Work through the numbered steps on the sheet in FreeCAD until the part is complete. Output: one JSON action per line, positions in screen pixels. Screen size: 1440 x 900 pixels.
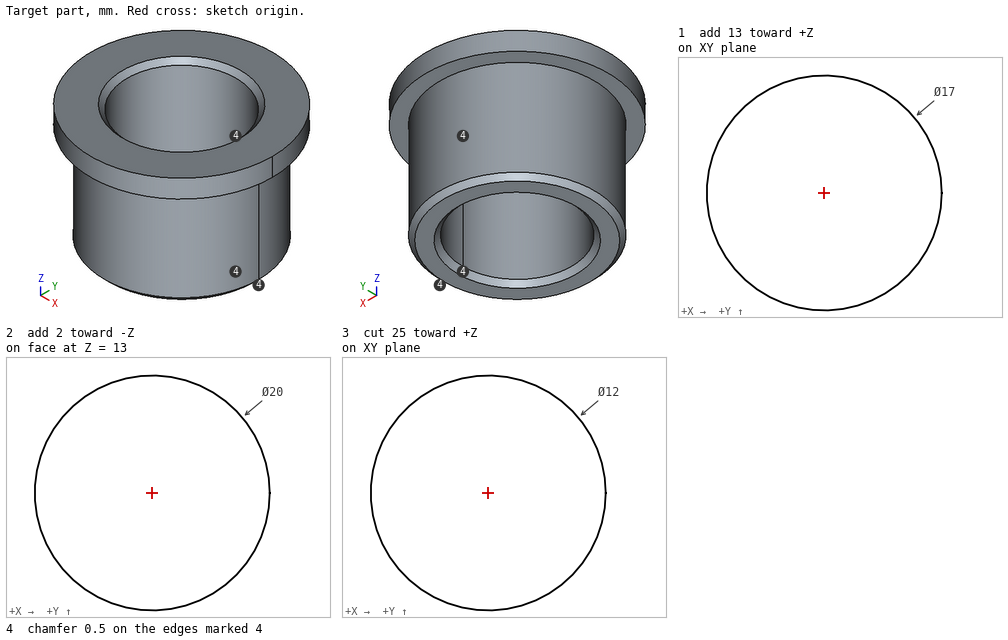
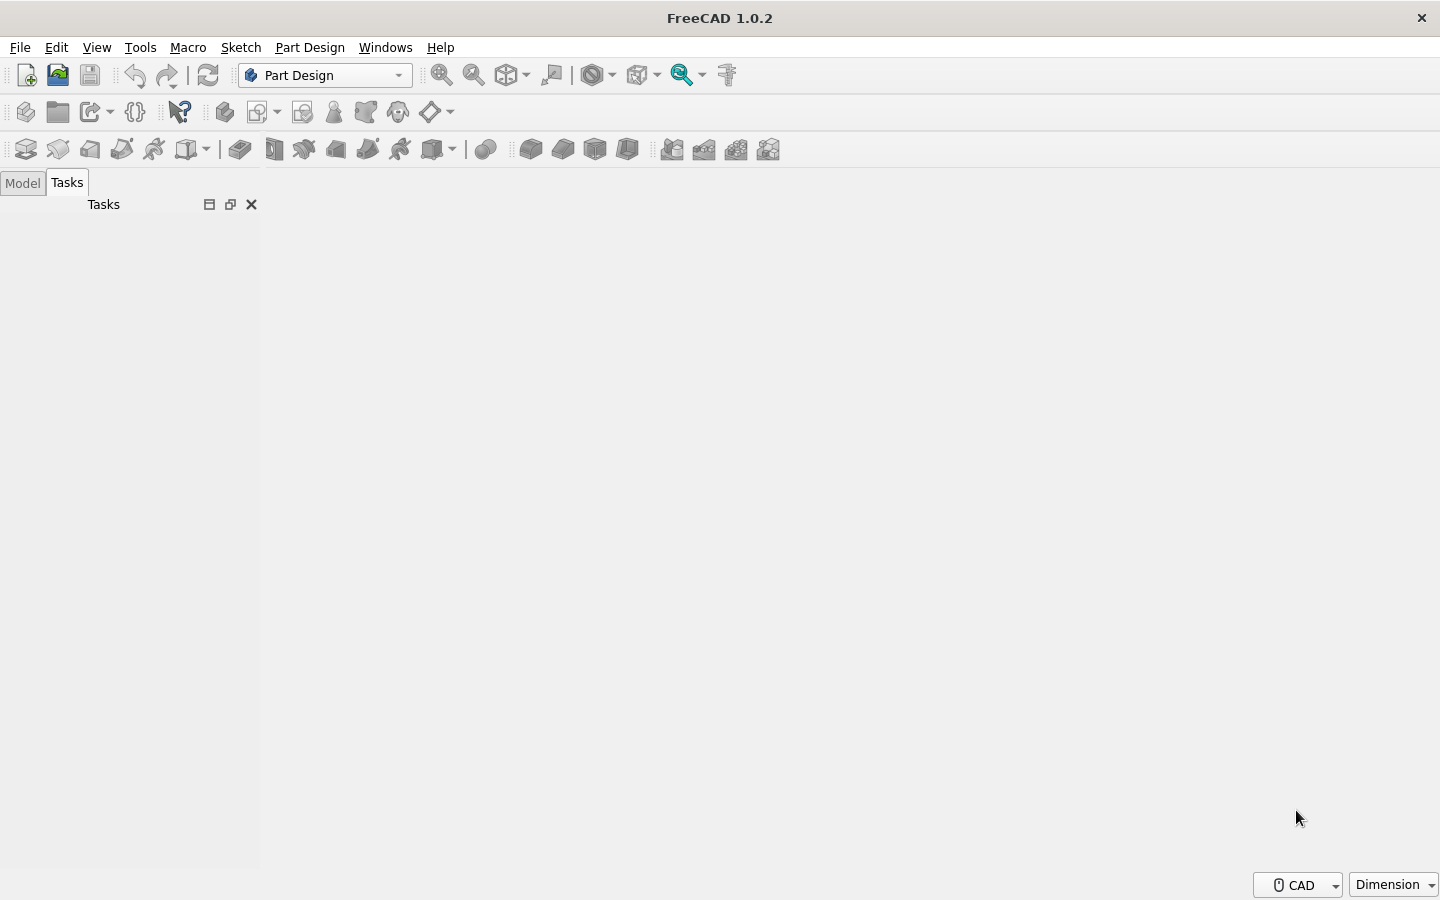
{"action": "left_click", "coordinate": [950, 76]}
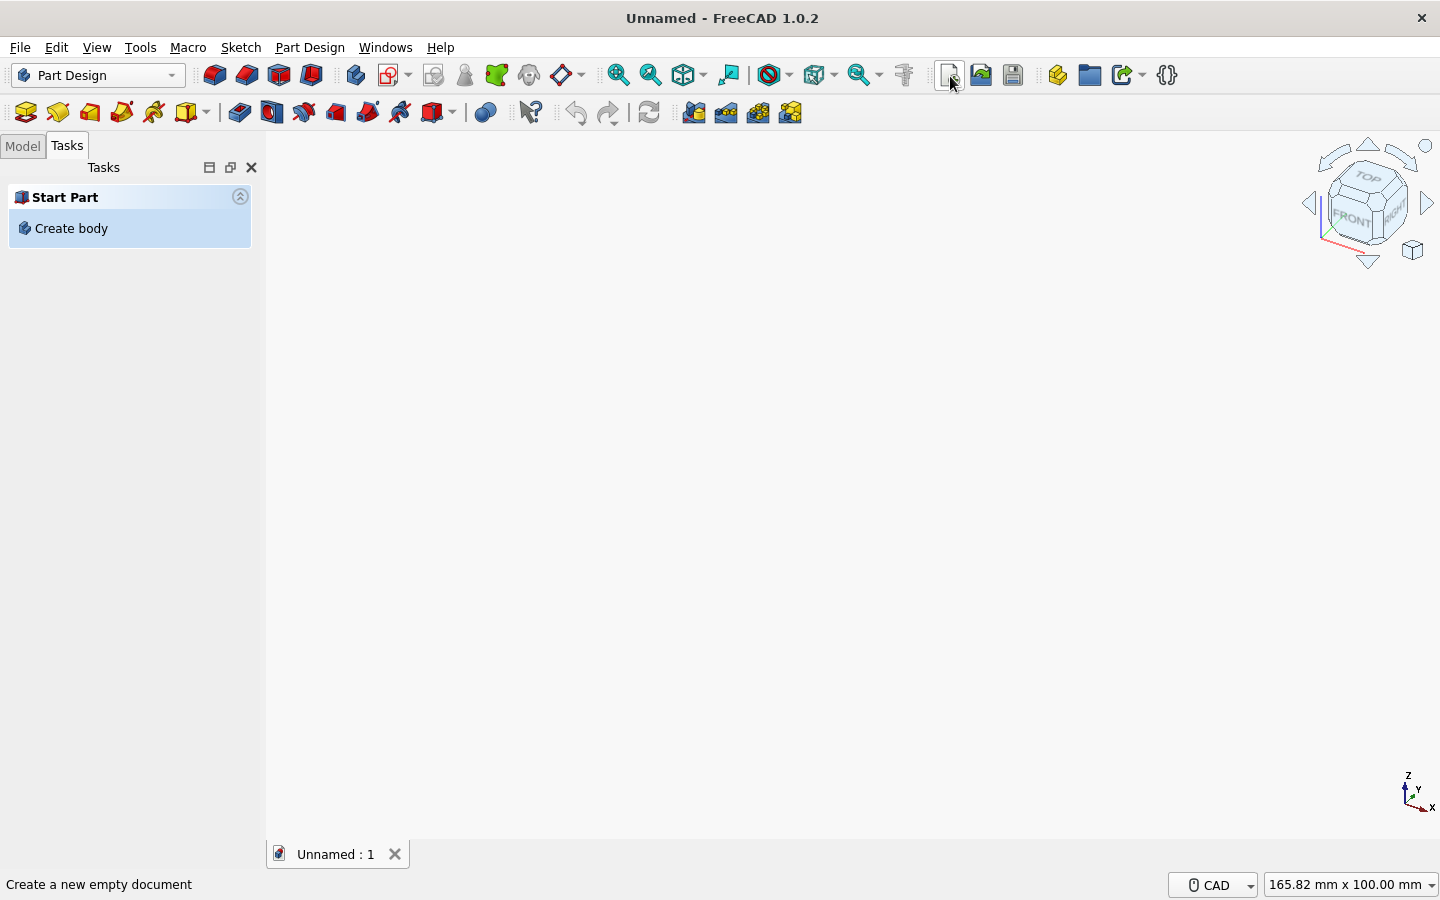
{"action": "left_click", "coordinate": [388, 76]}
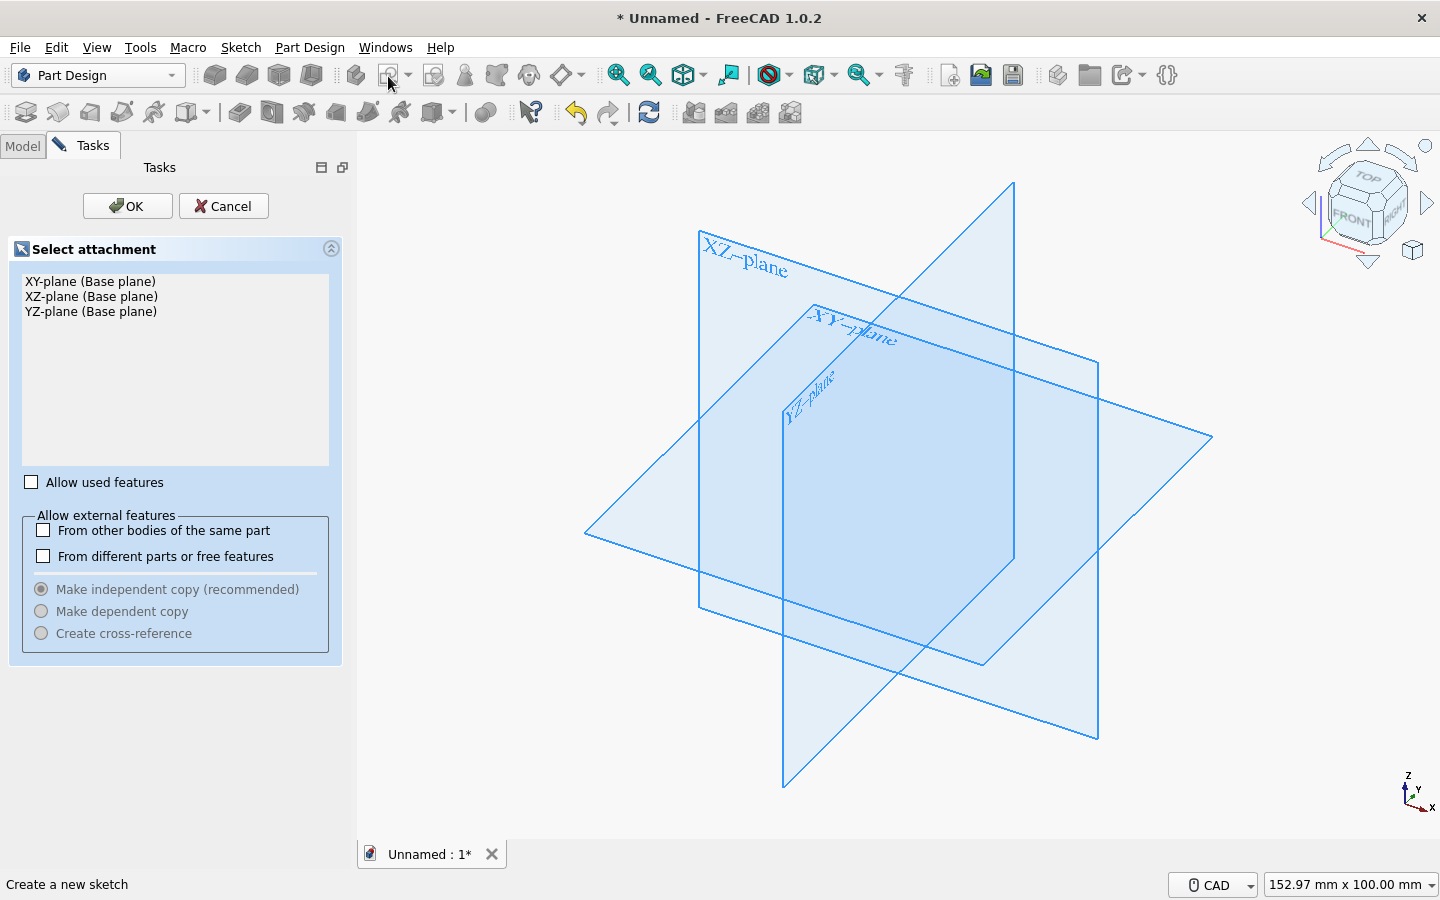
{"action": "left_click", "coordinate": [82, 282]}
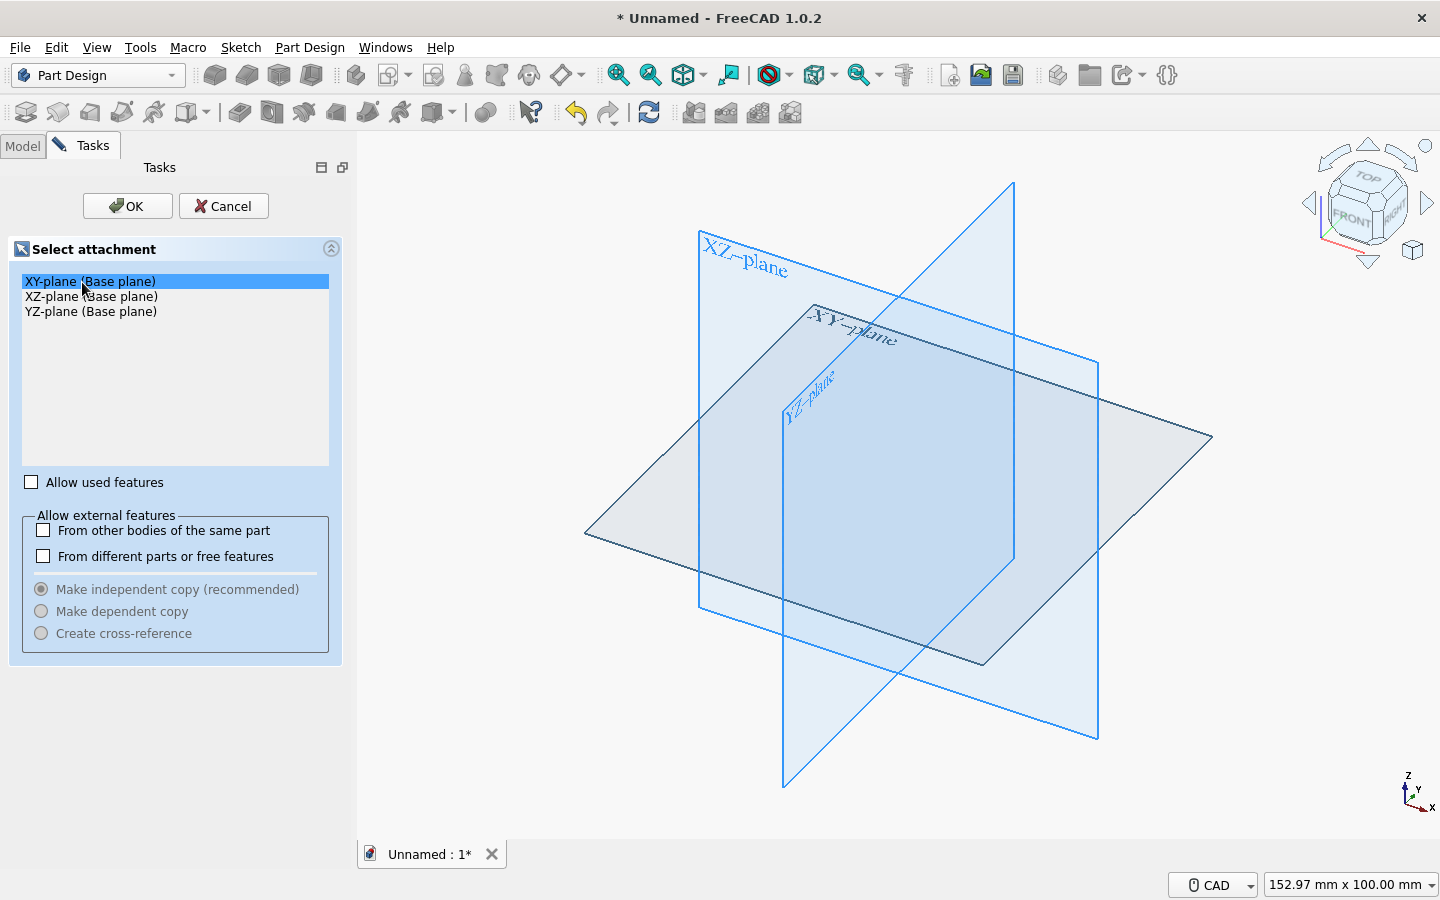
{"action": "left_click", "coordinate": [128, 206]}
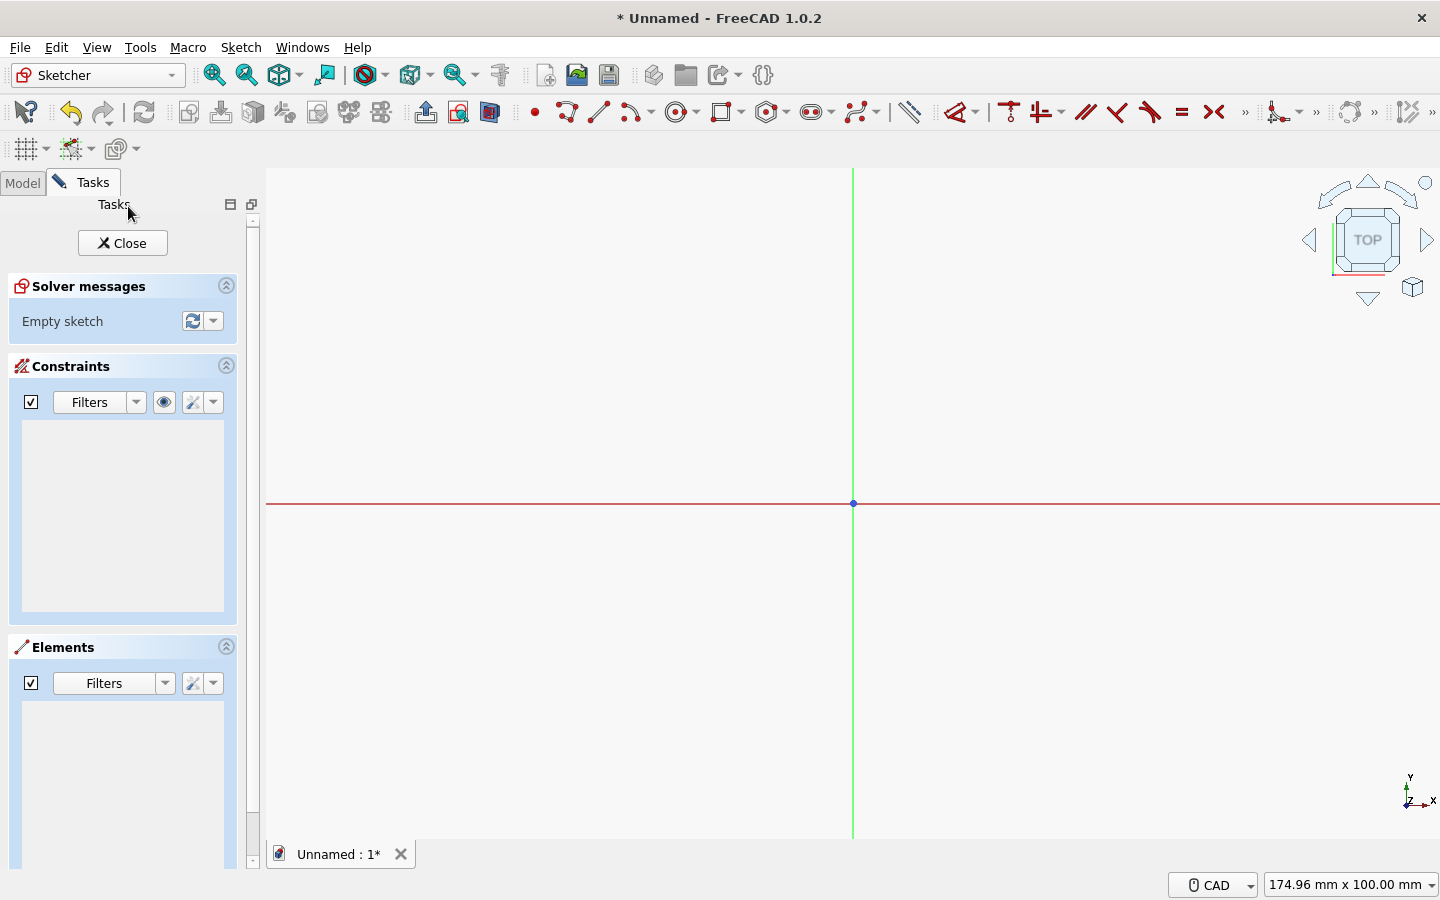
{"action": "scroll", "coordinate": [875, 504], "scroll_direction": "up", "scroll_amount": 7}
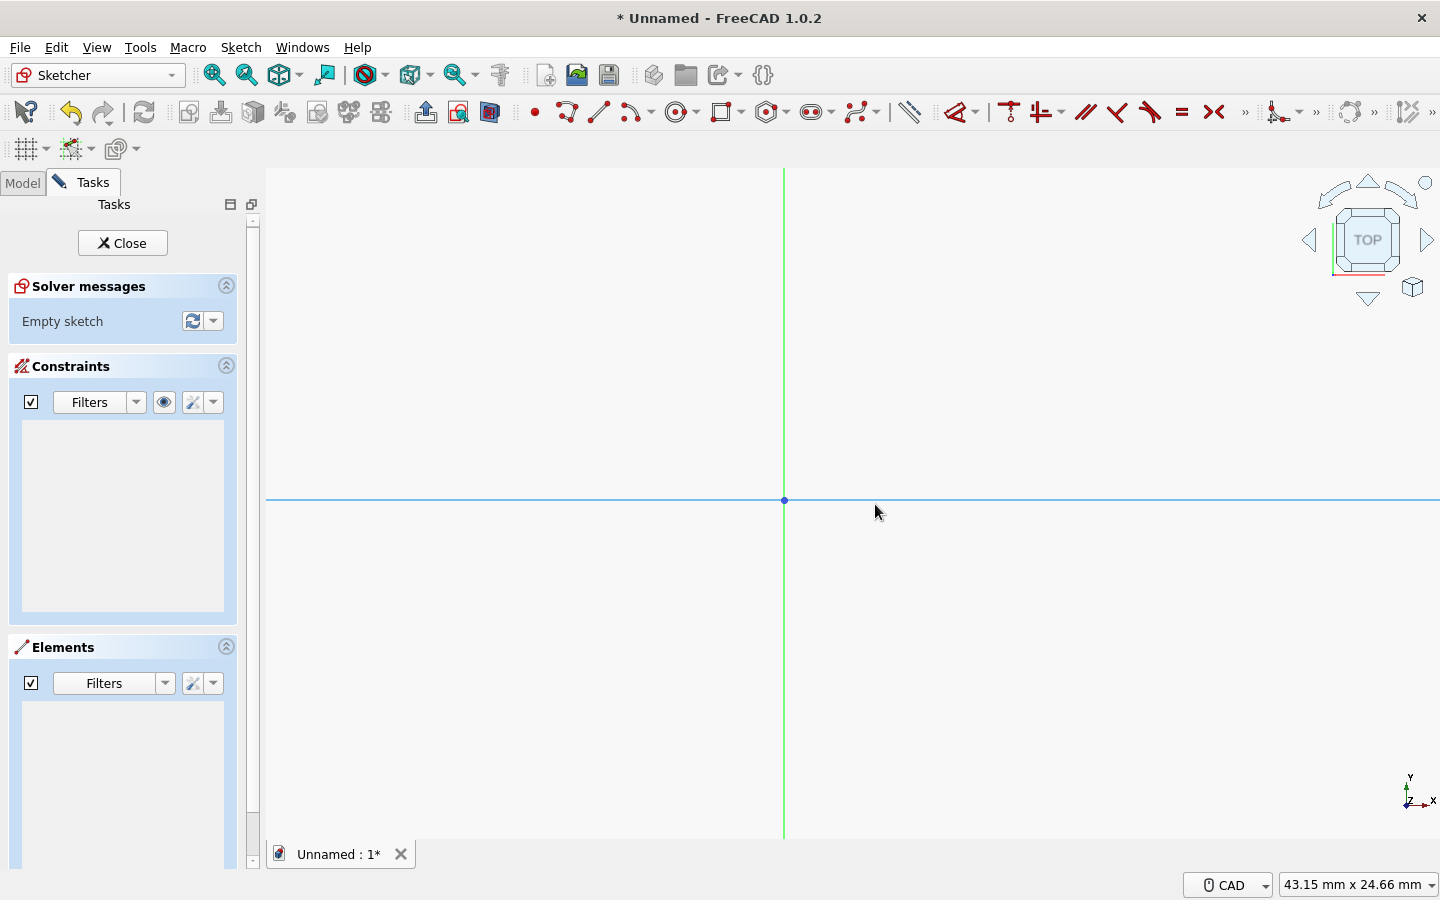
{"action": "key", "text": "g c"}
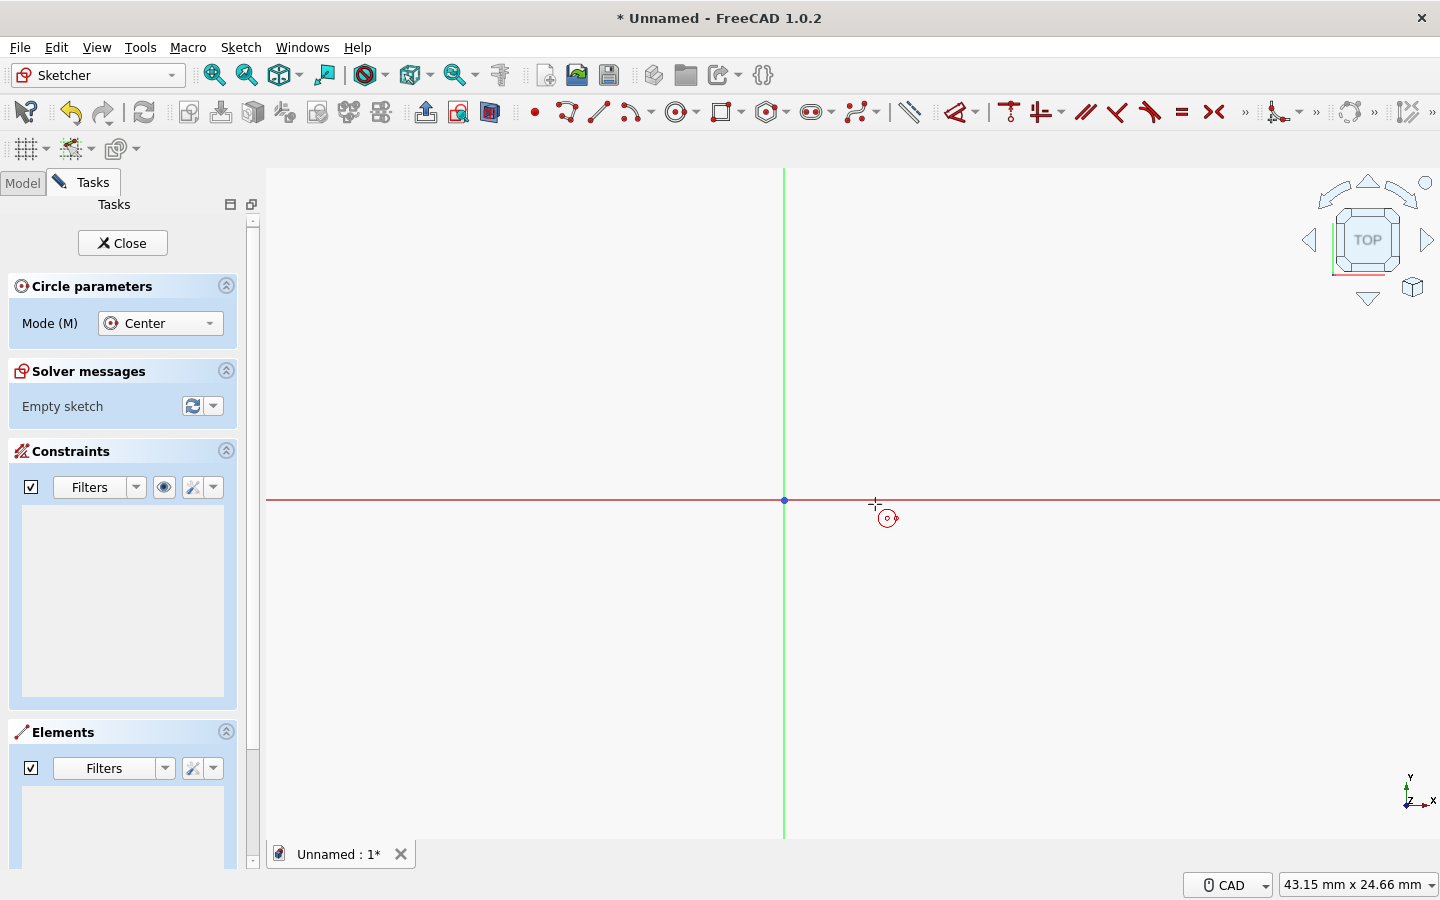
{"action": "left_click", "coordinate": [784, 500]}
{"action": "left_click", "coordinate": [948, 337]}
{"action": "key", "text": "Escape"}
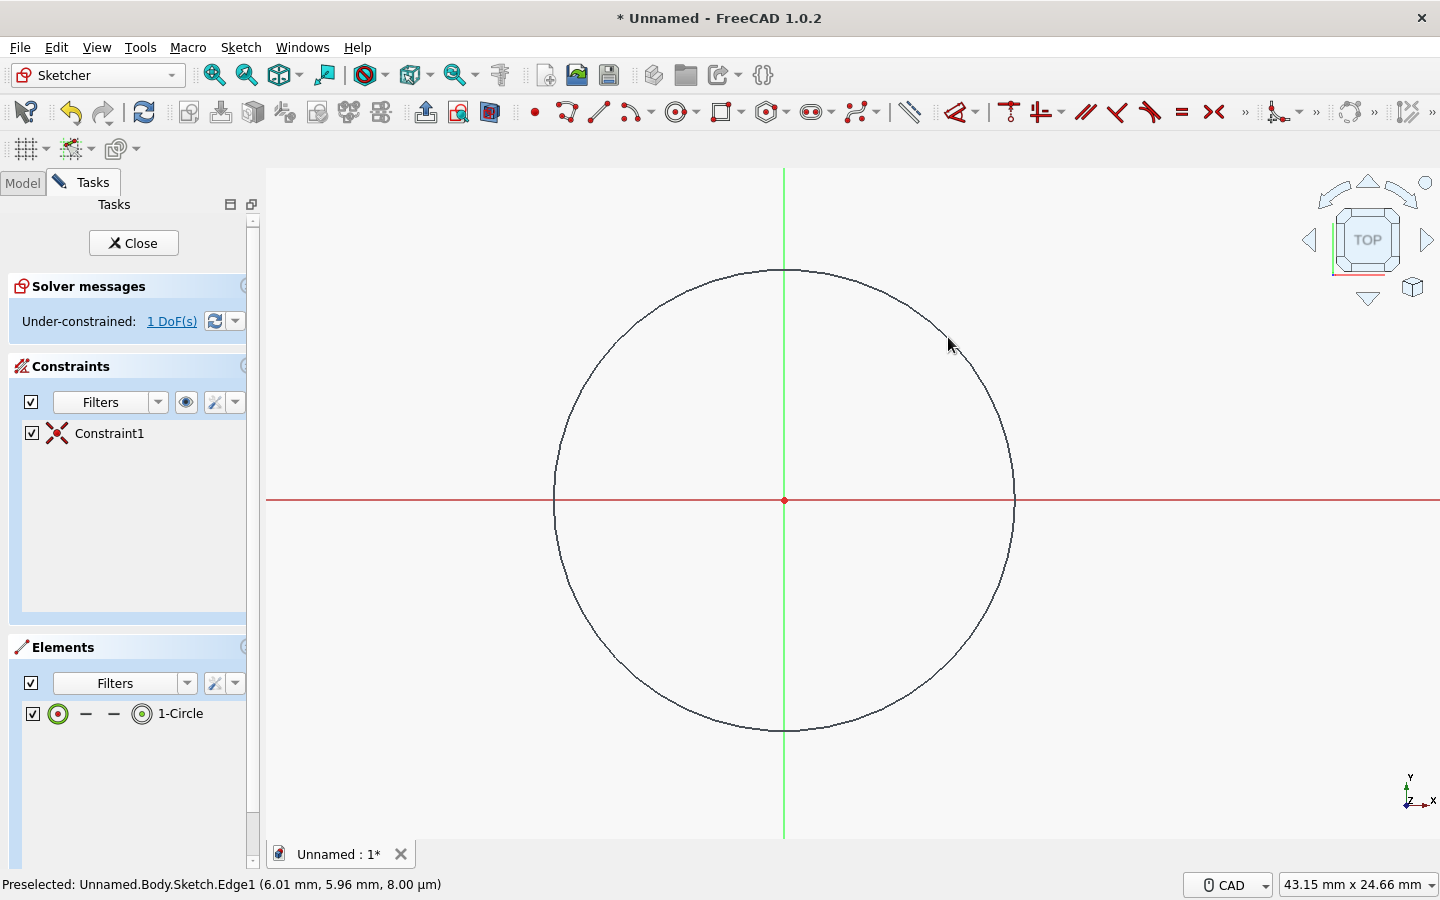
{"action": "left_click", "coordinate": [947, 337]}